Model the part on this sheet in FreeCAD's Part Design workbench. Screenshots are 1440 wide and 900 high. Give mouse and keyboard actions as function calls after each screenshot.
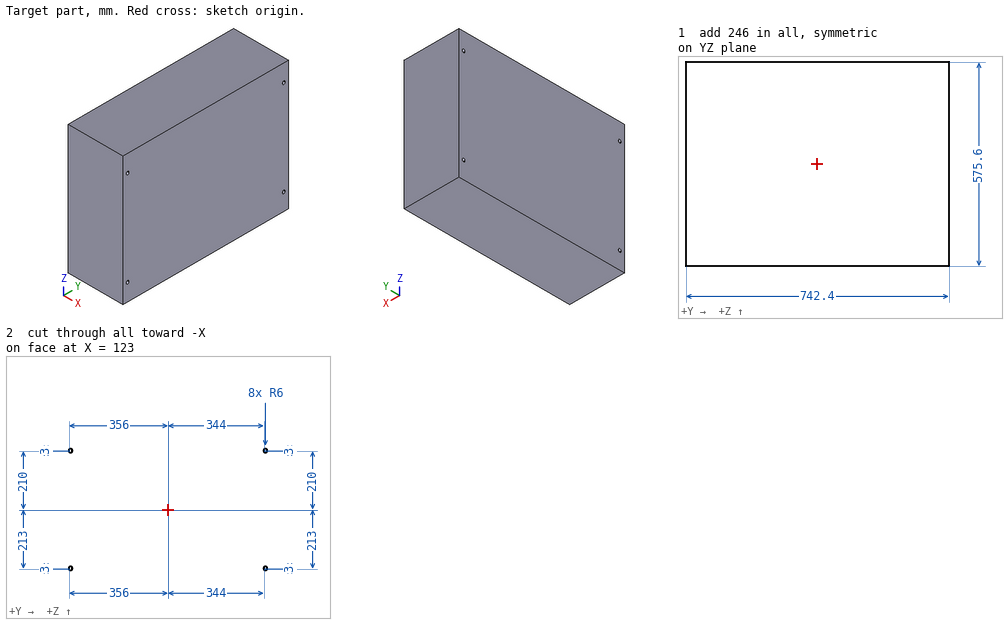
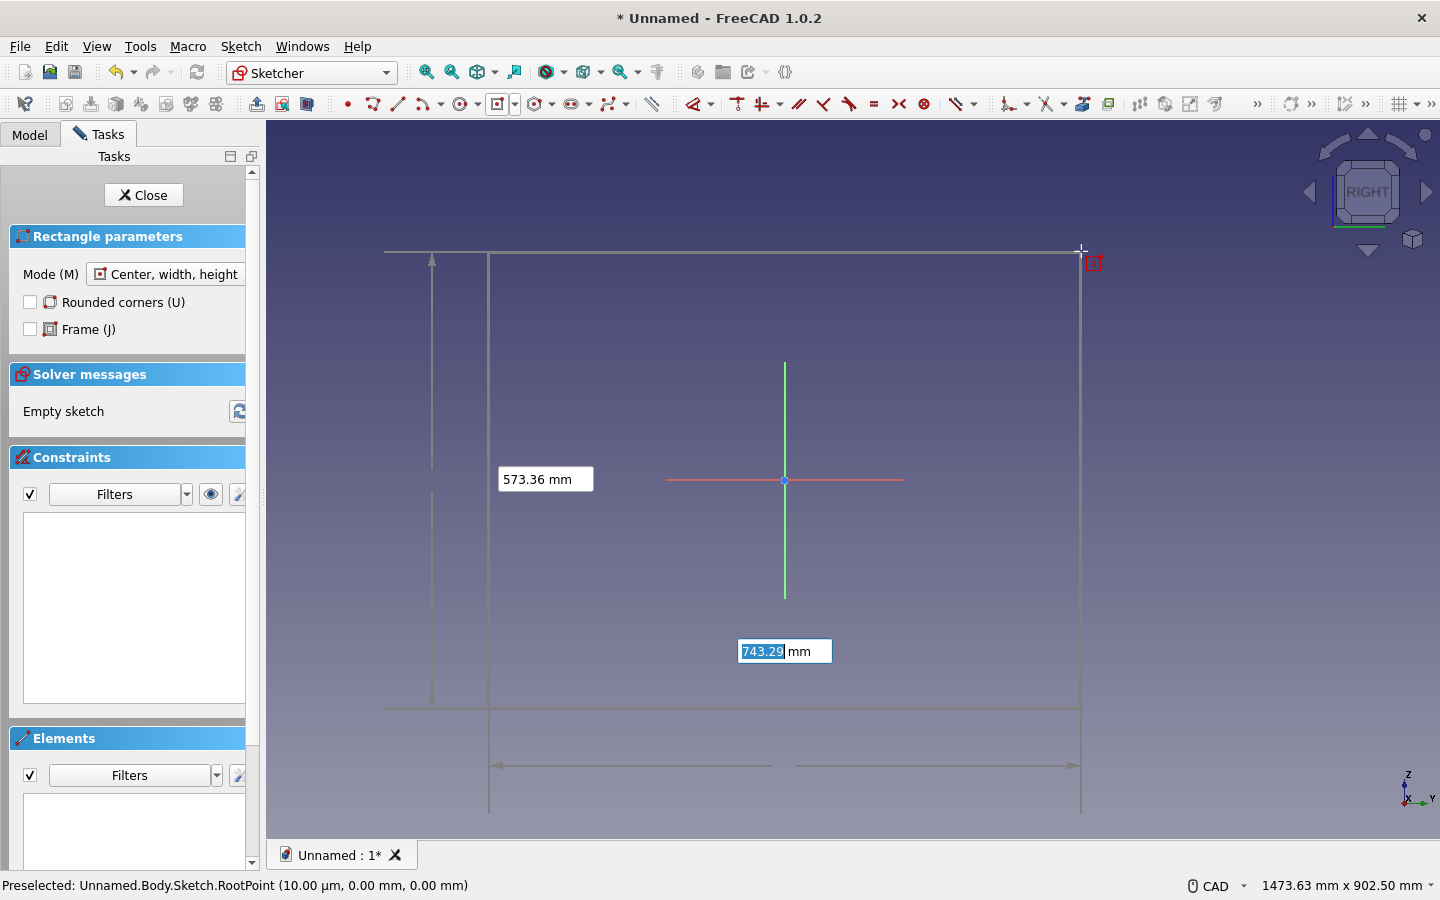
text(742.4)
key(Tab)
text(575.6)
key(Return)
key(Escape)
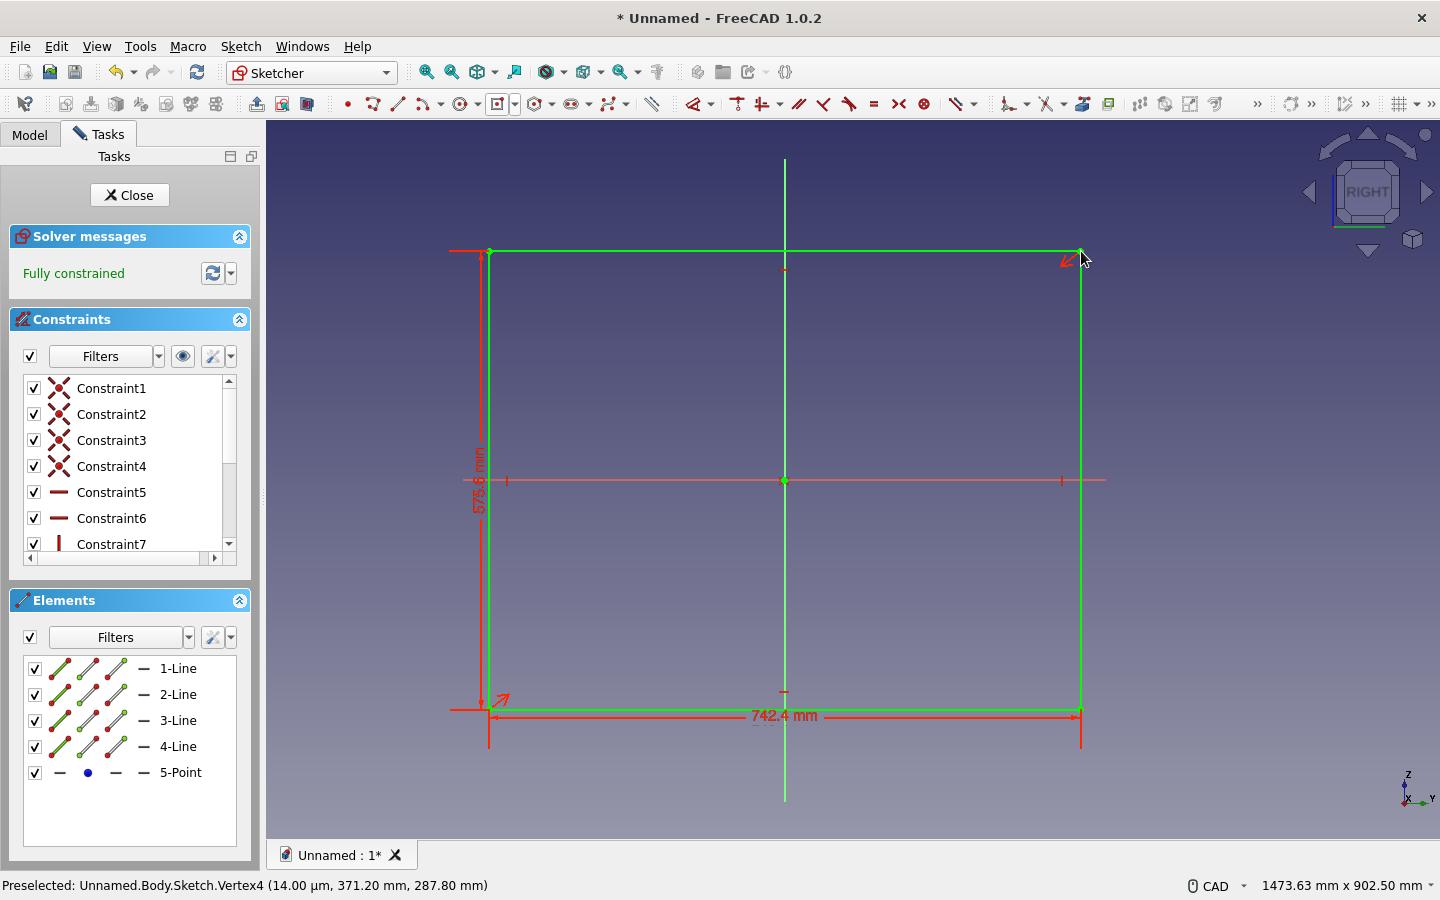
click(130, 195)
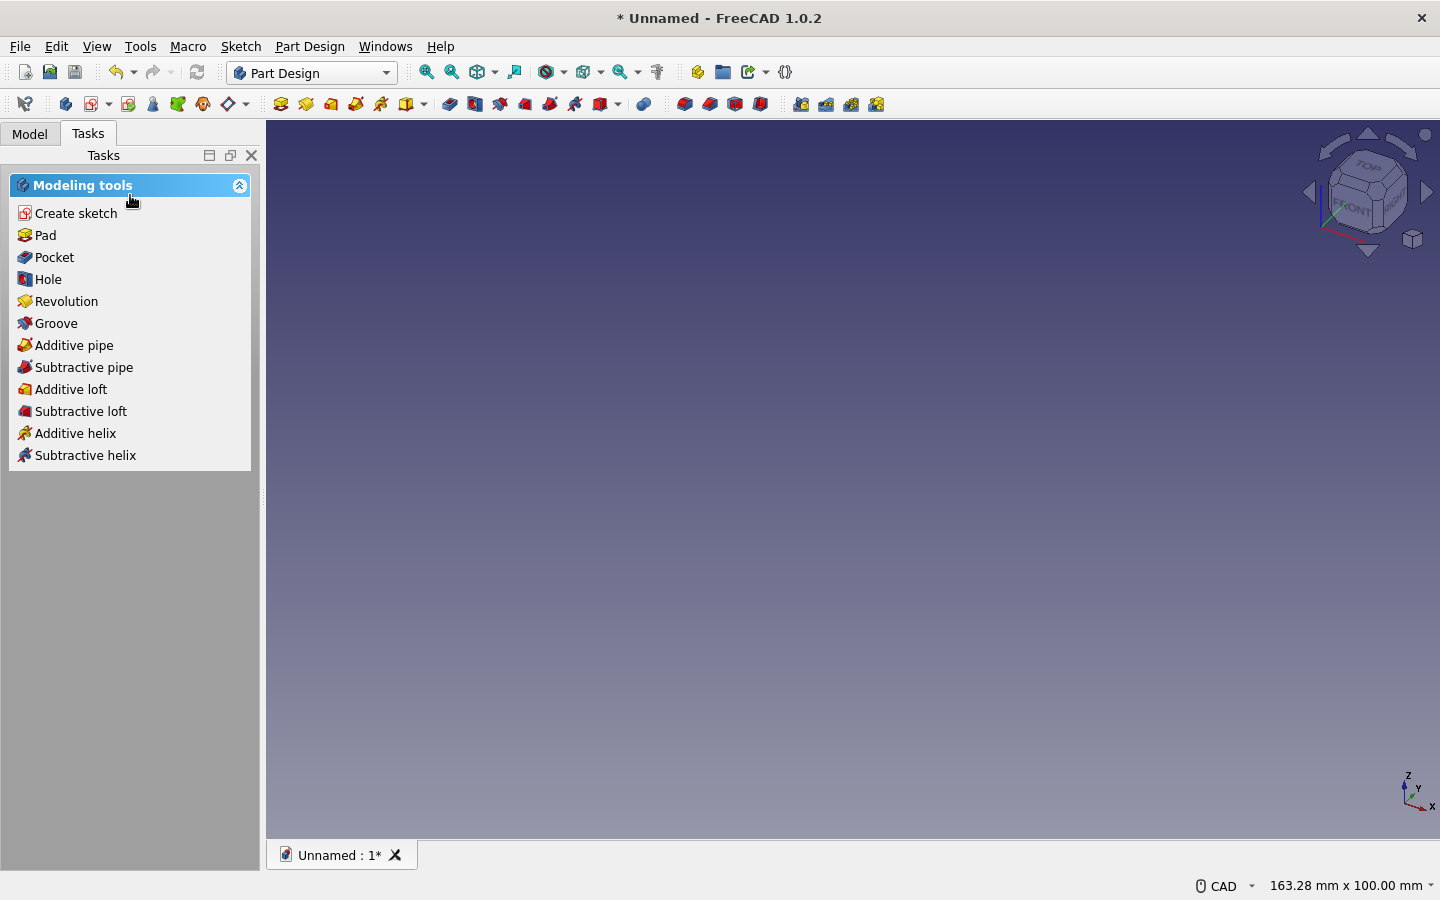
click(281, 104)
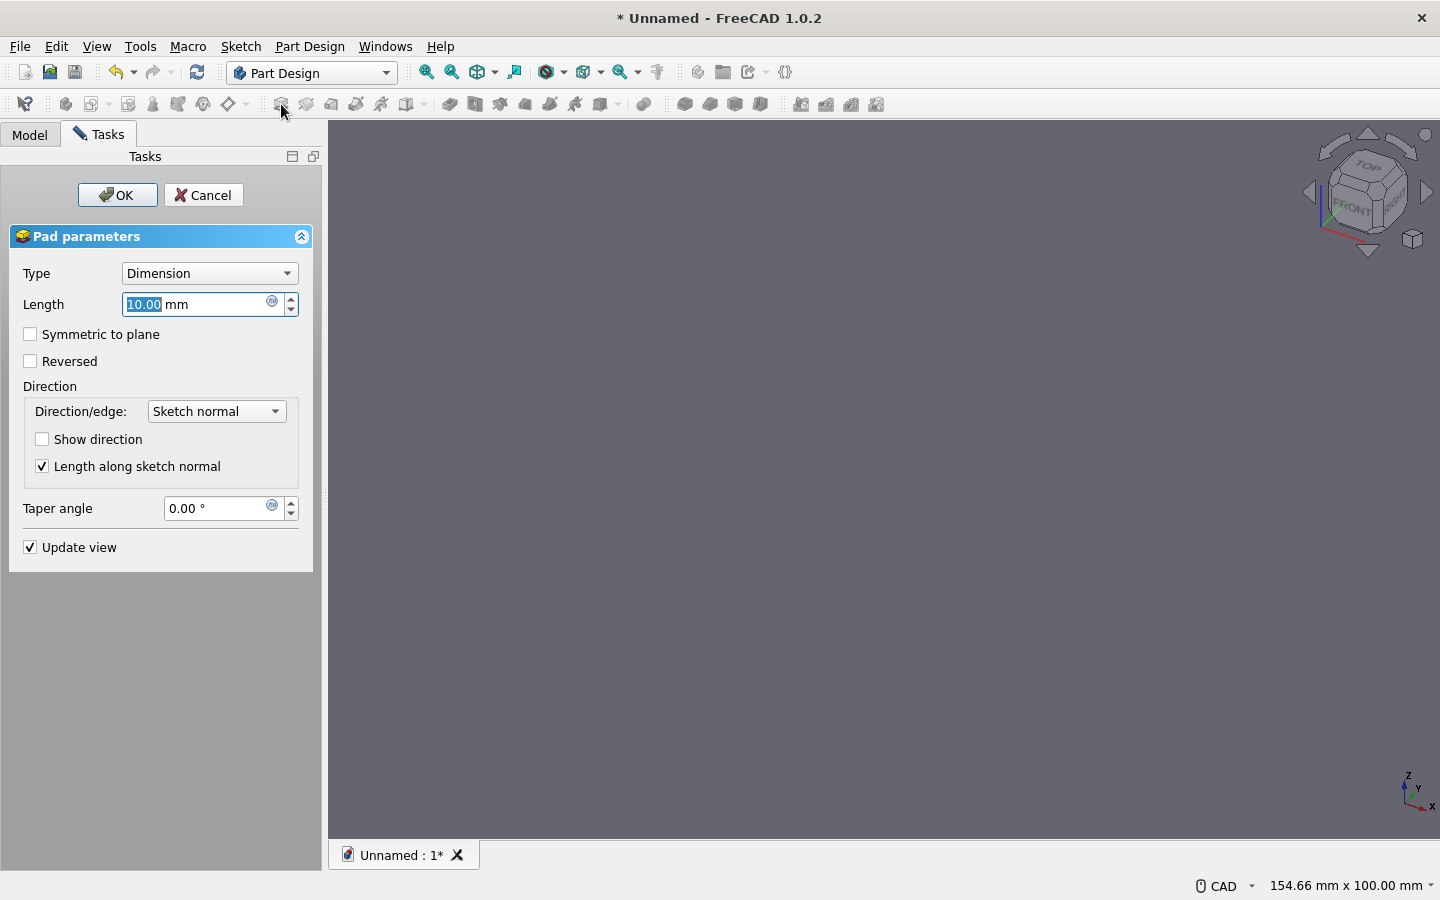
text(246)
key(Tab)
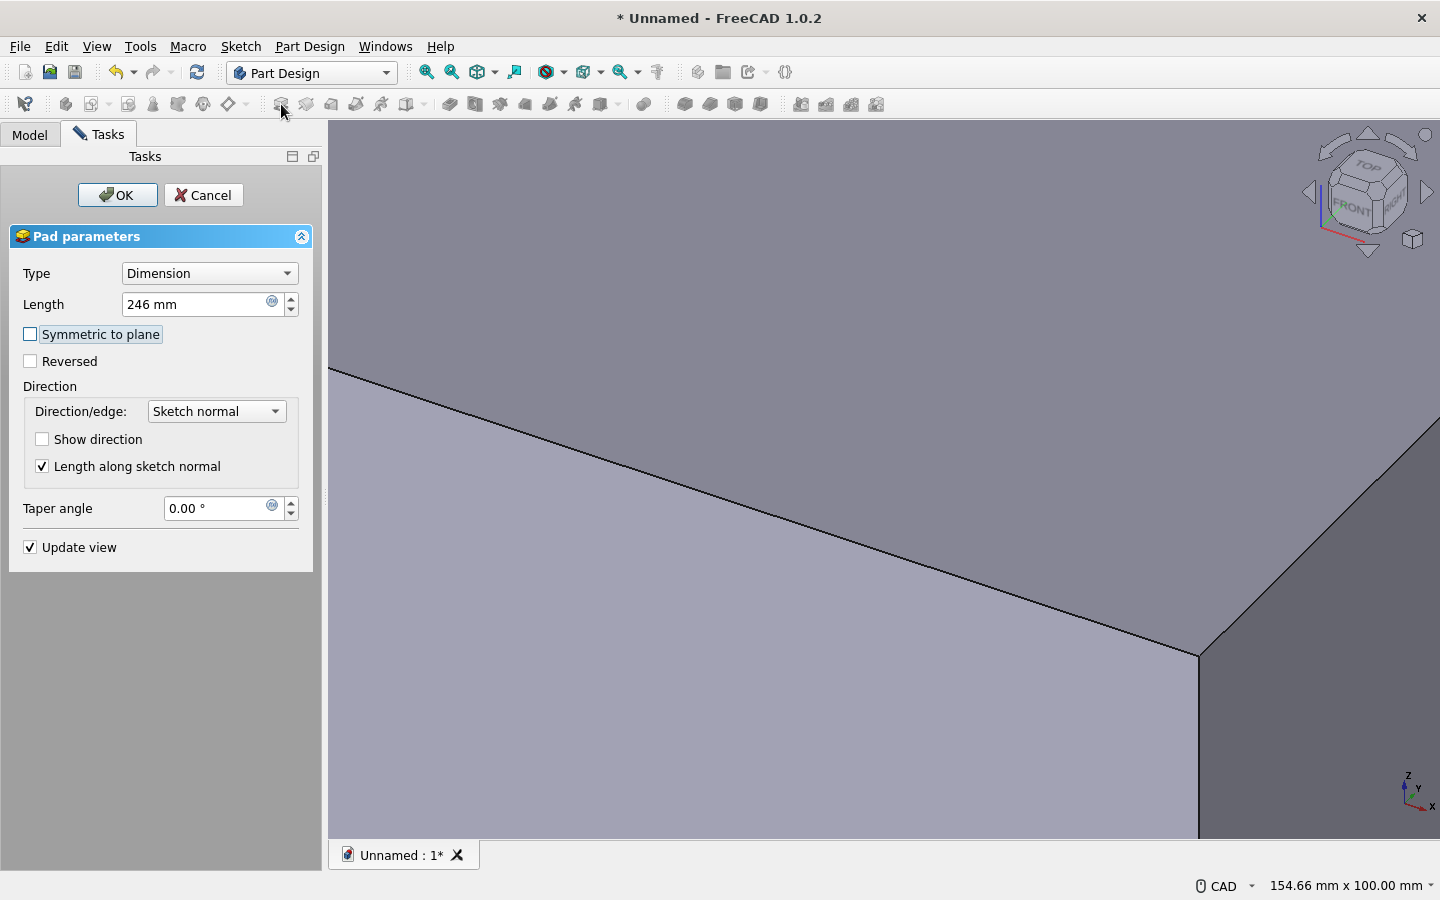
click(31, 334)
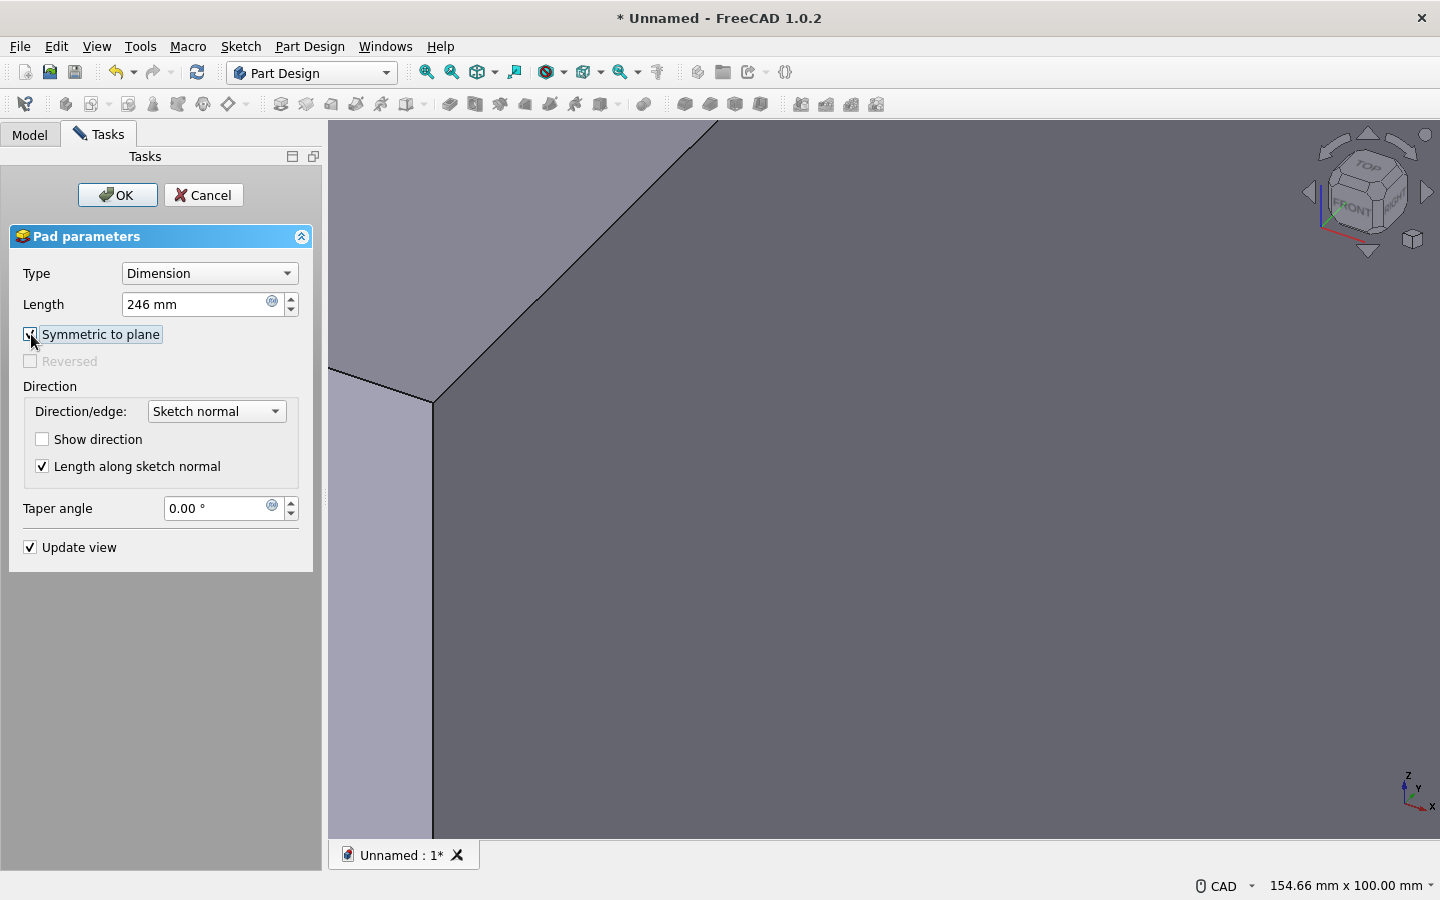
click(118, 195)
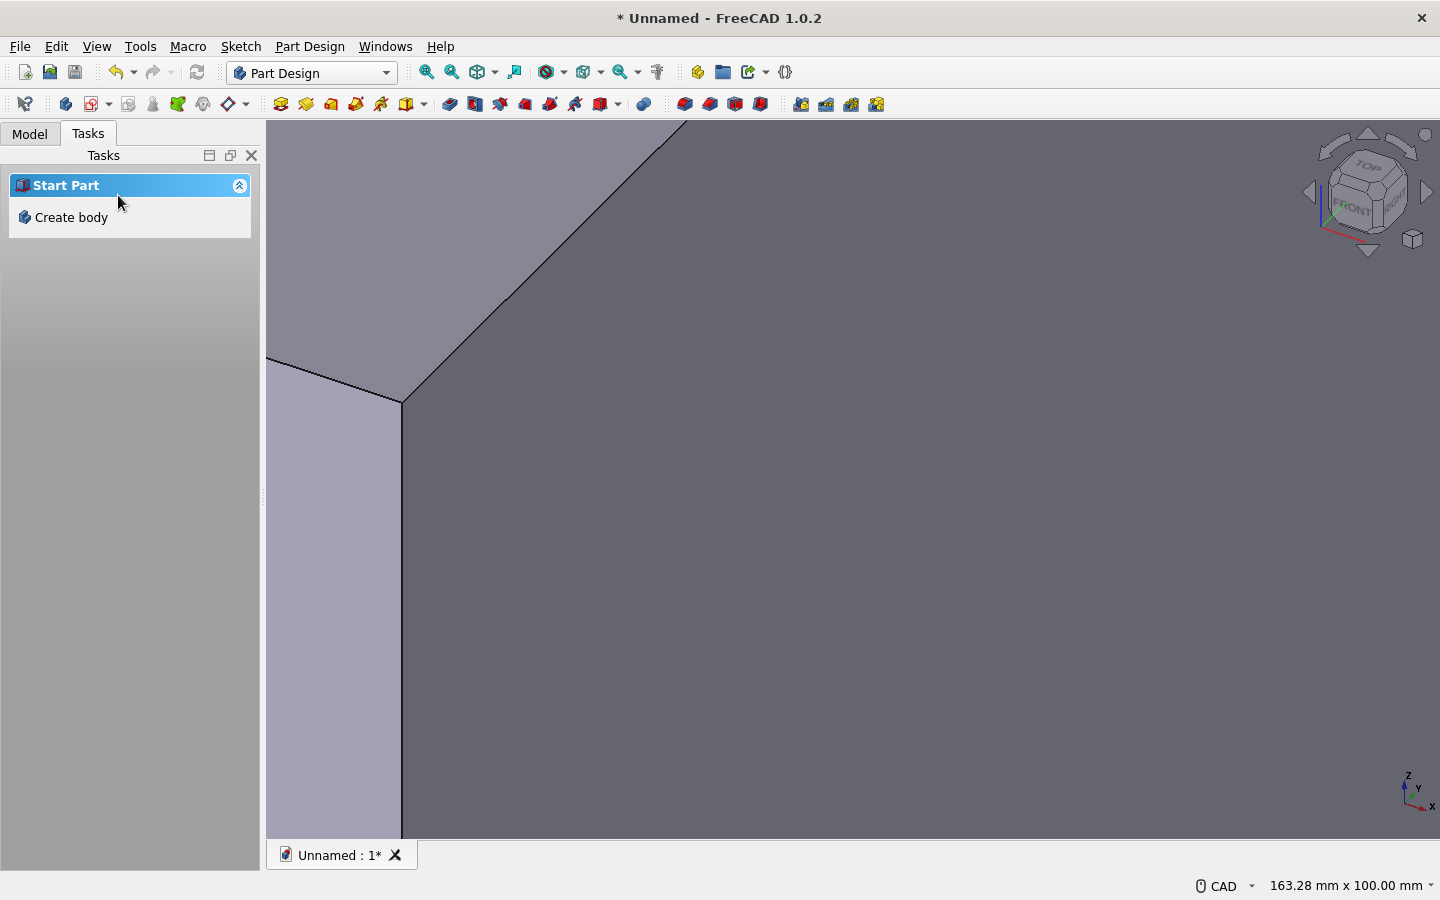
click(427, 72)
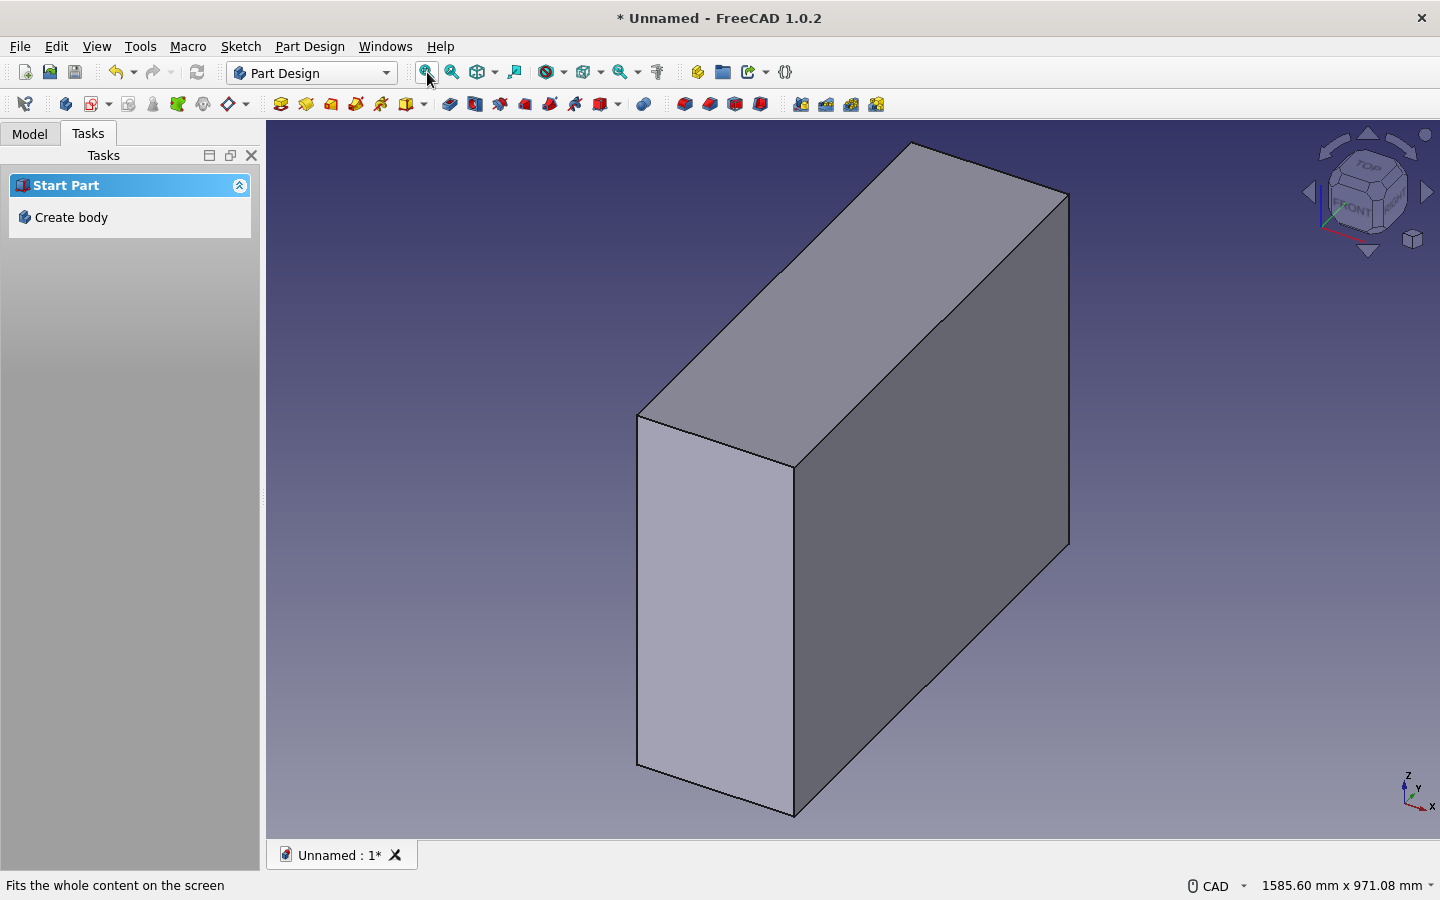
click(932, 505)